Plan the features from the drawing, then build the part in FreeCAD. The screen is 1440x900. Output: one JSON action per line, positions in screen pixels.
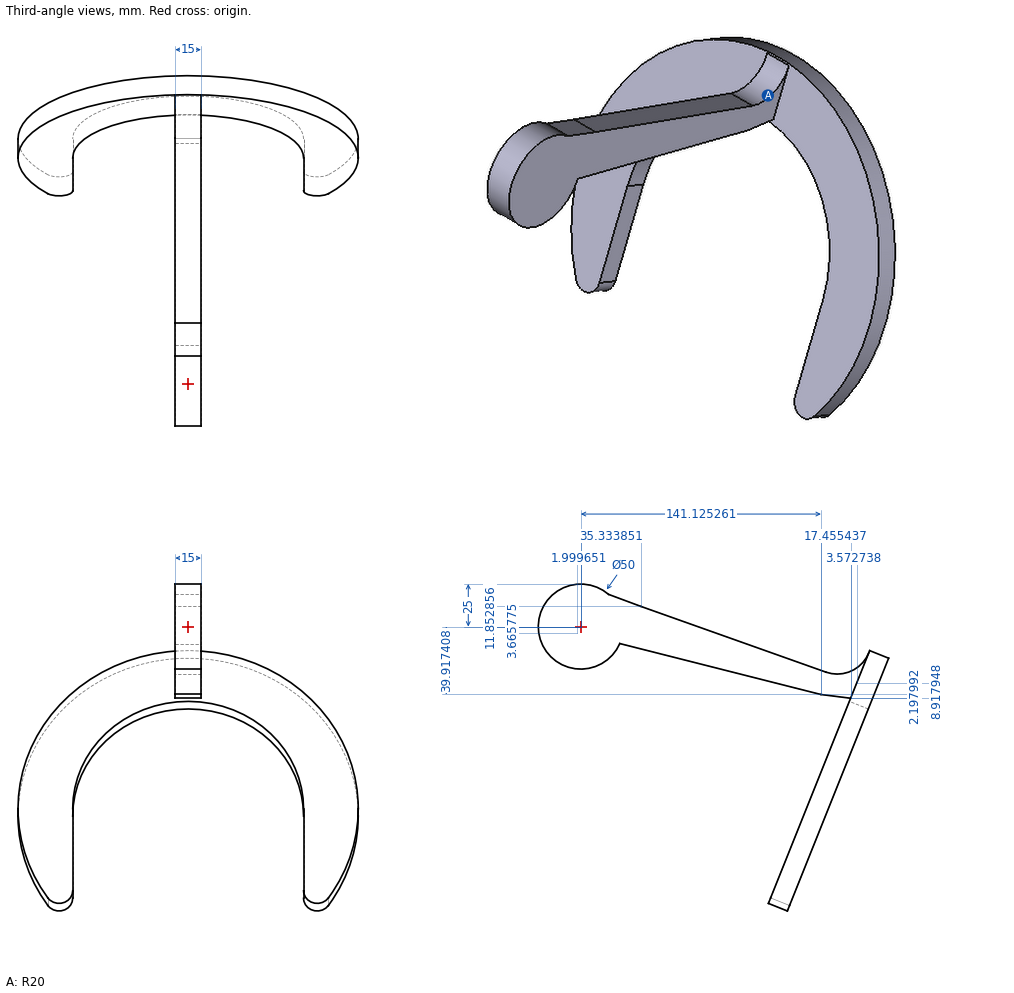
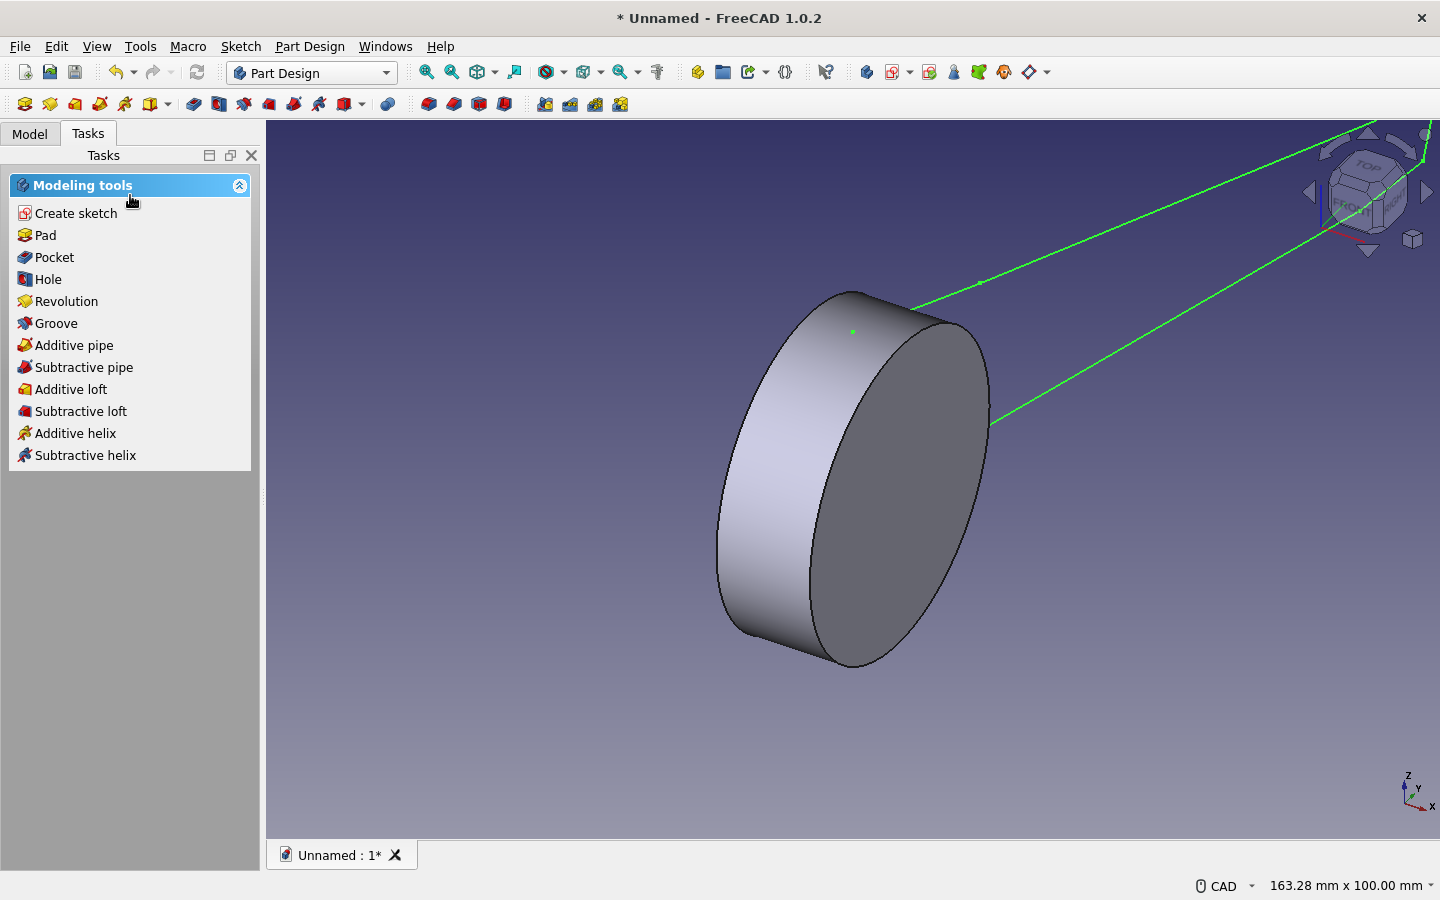
{"action": "left_click", "coordinate": [25, 104]}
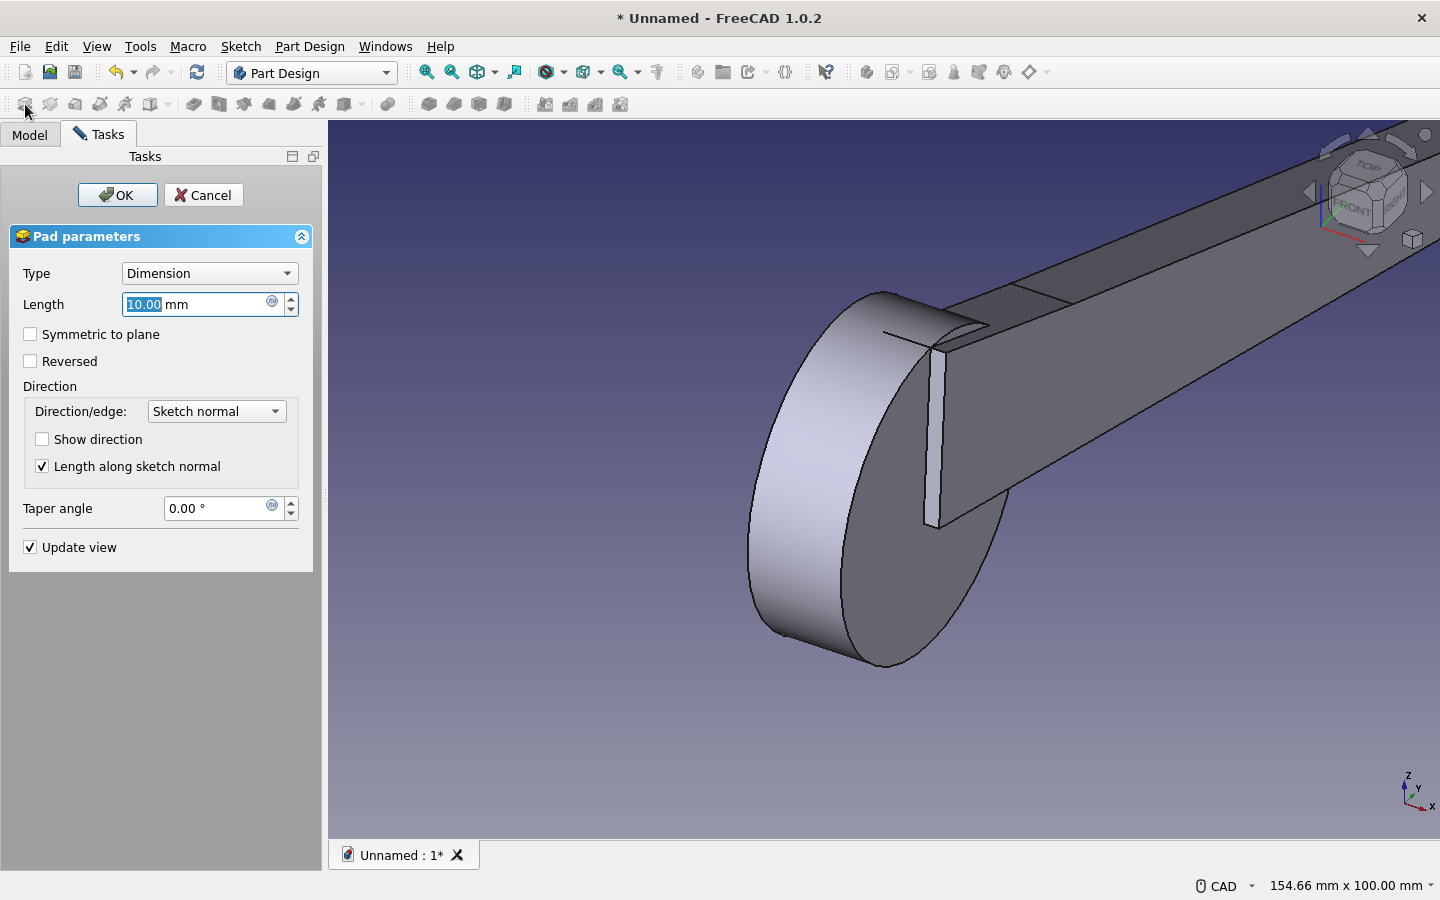
{"action": "type", "text": "15"}
{"action": "key", "text": "Tab"}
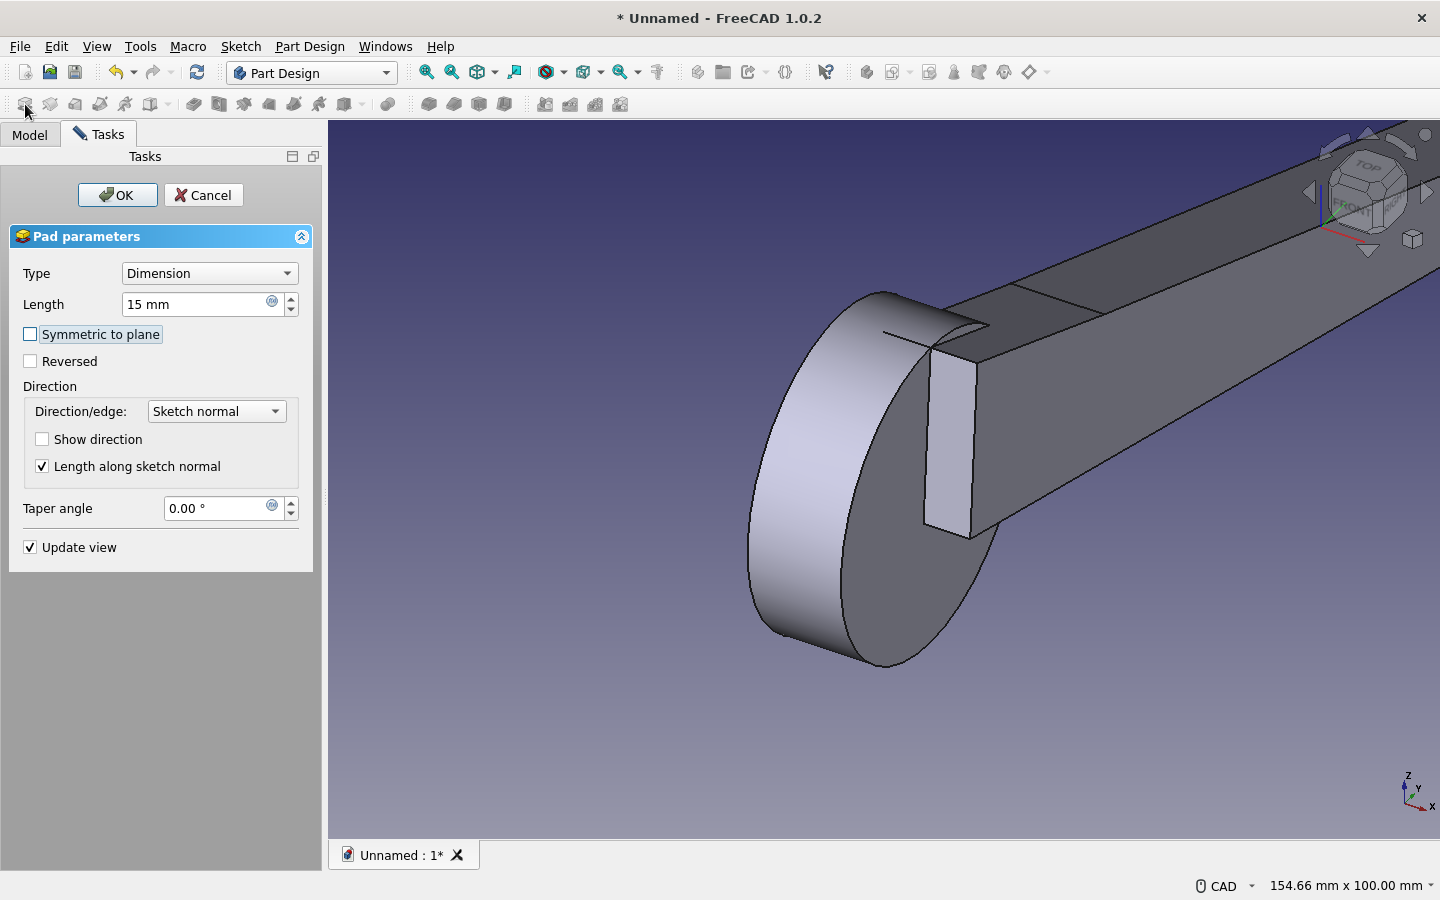
{"action": "left_click", "coordinate": [31, 334]}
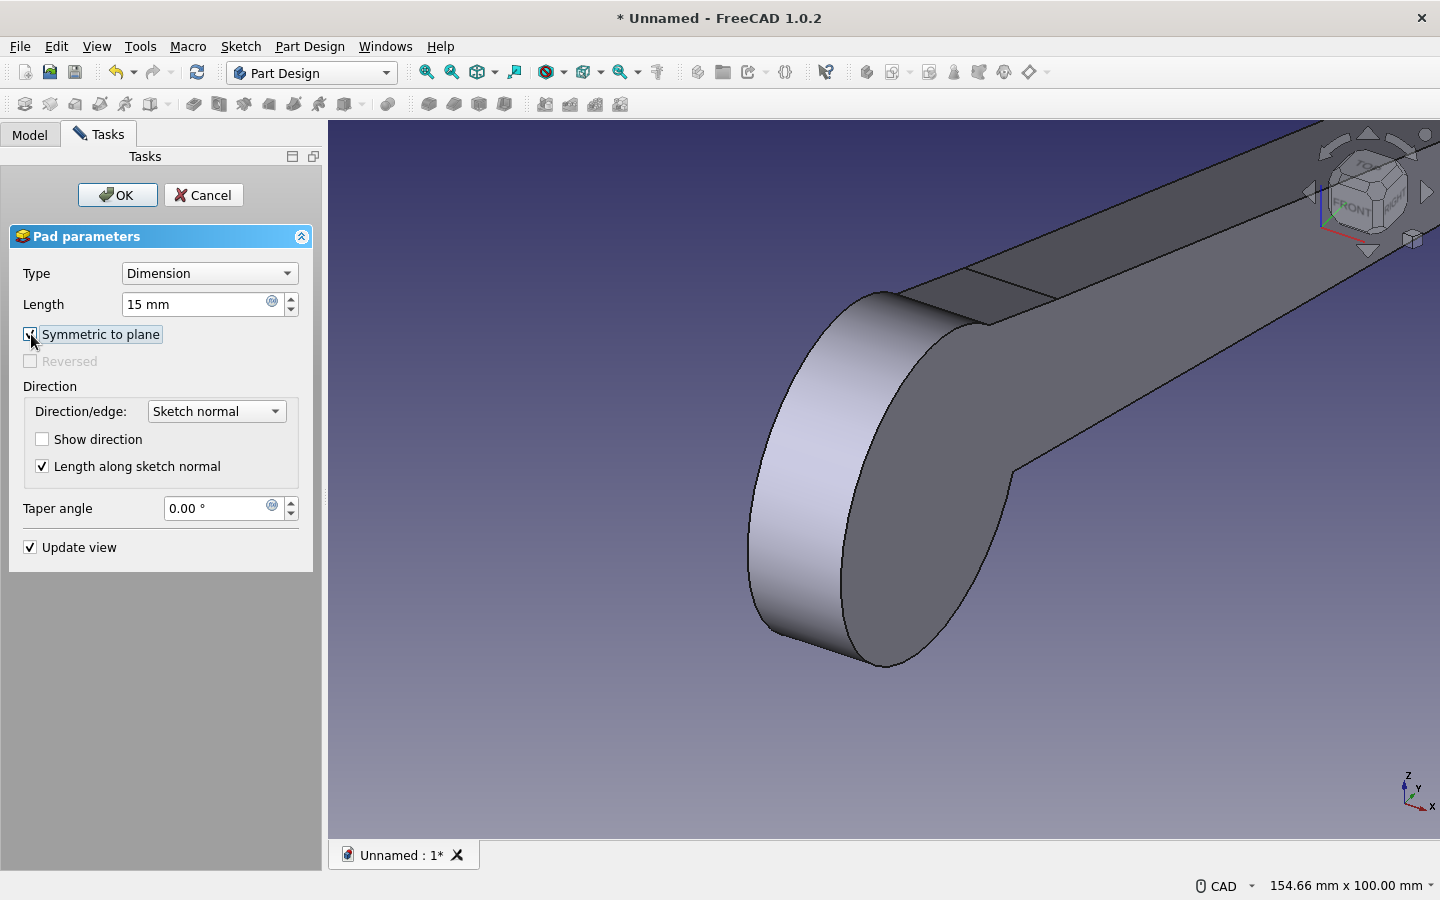
{"action": "left_click", "coordinate": [118, 195]}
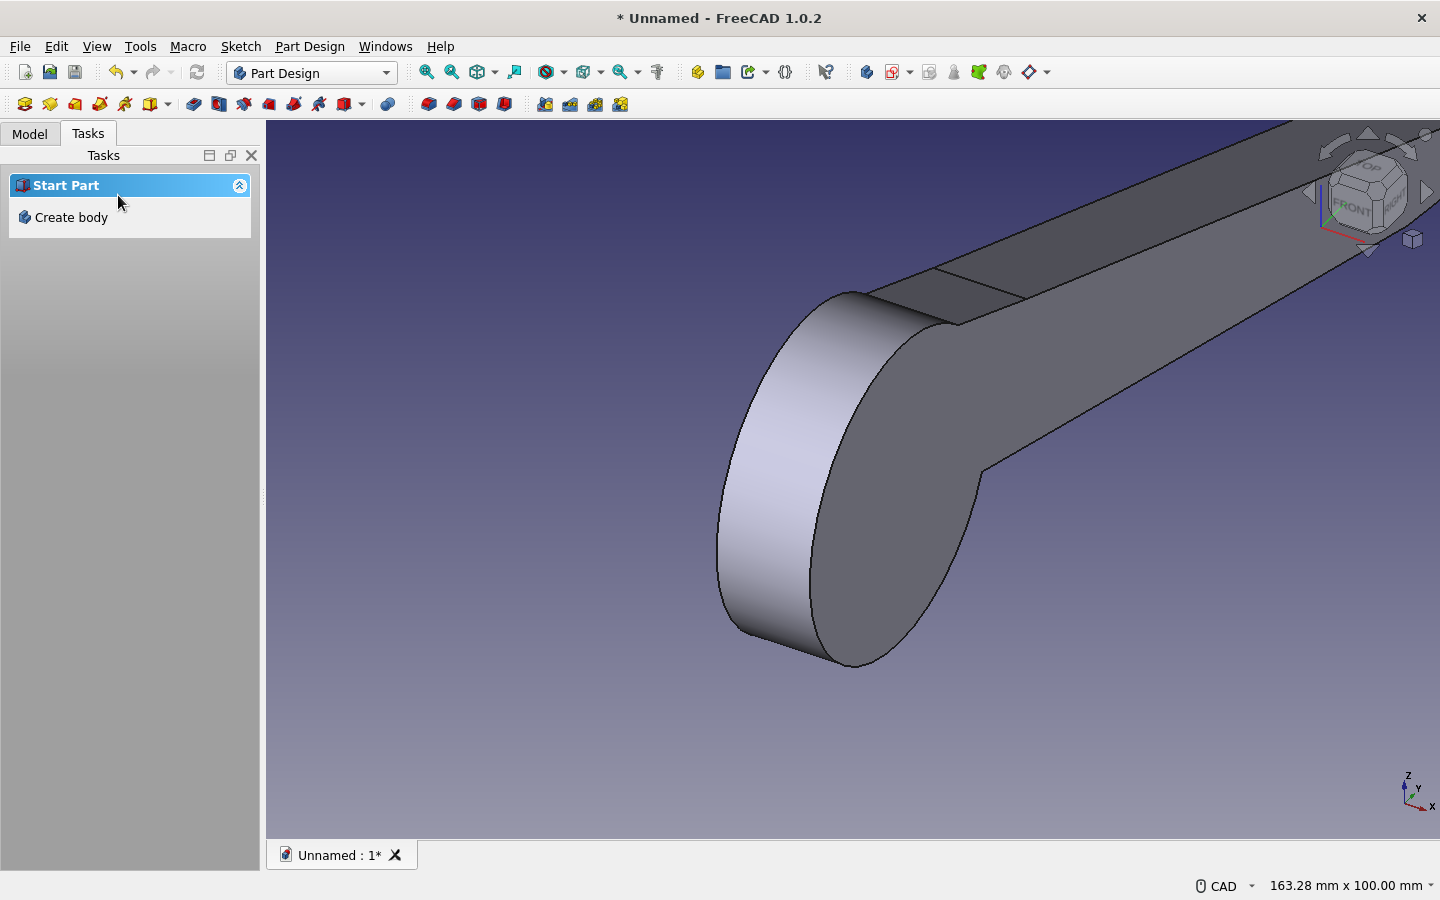
{"action": "left_click", "coordinate": [427, 72]}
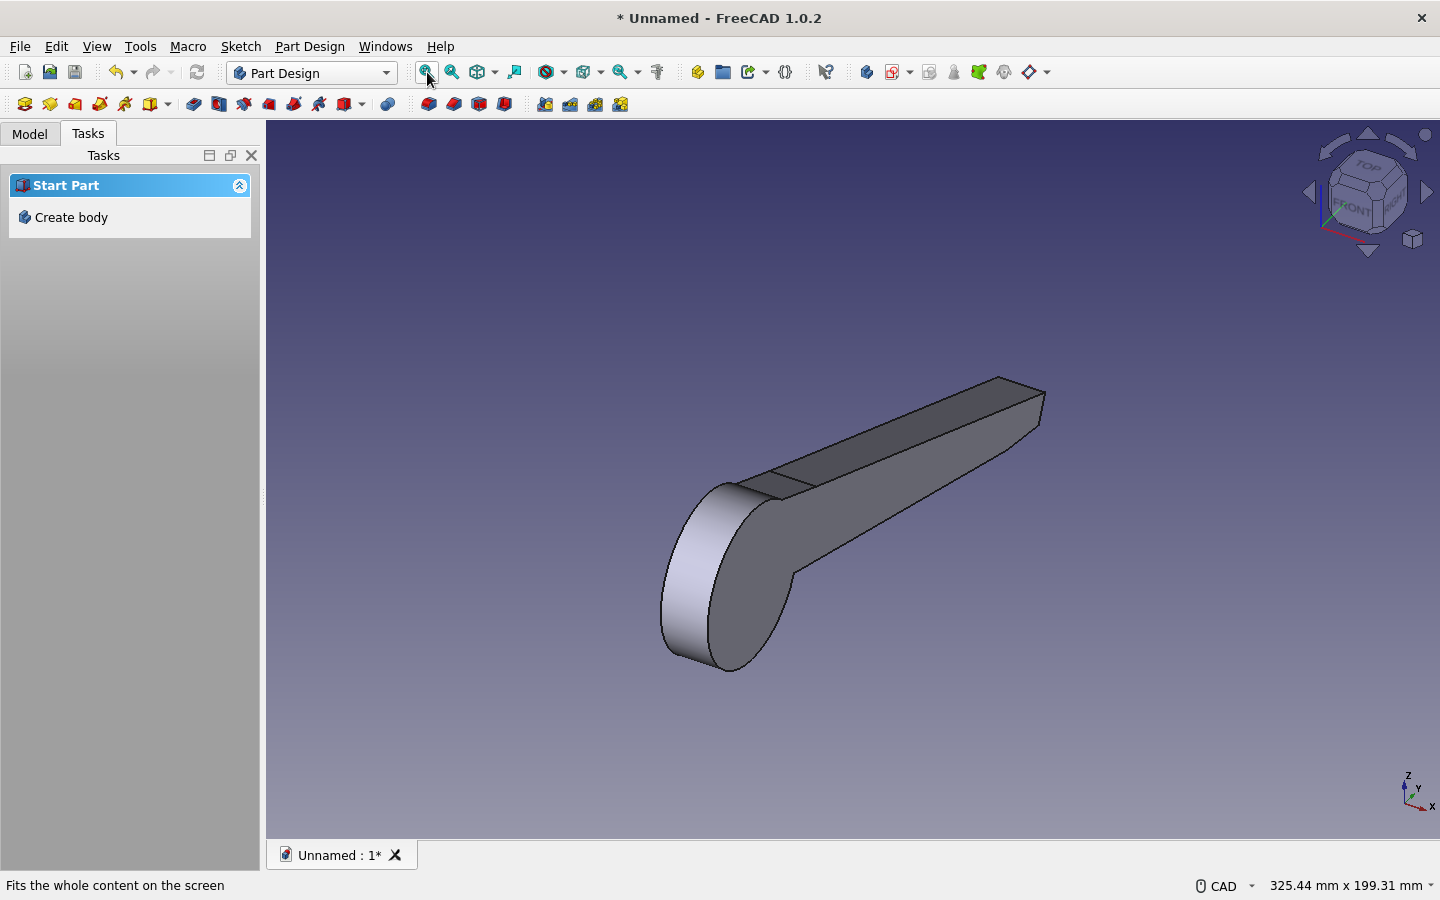
{"action": "key", "text": "4"}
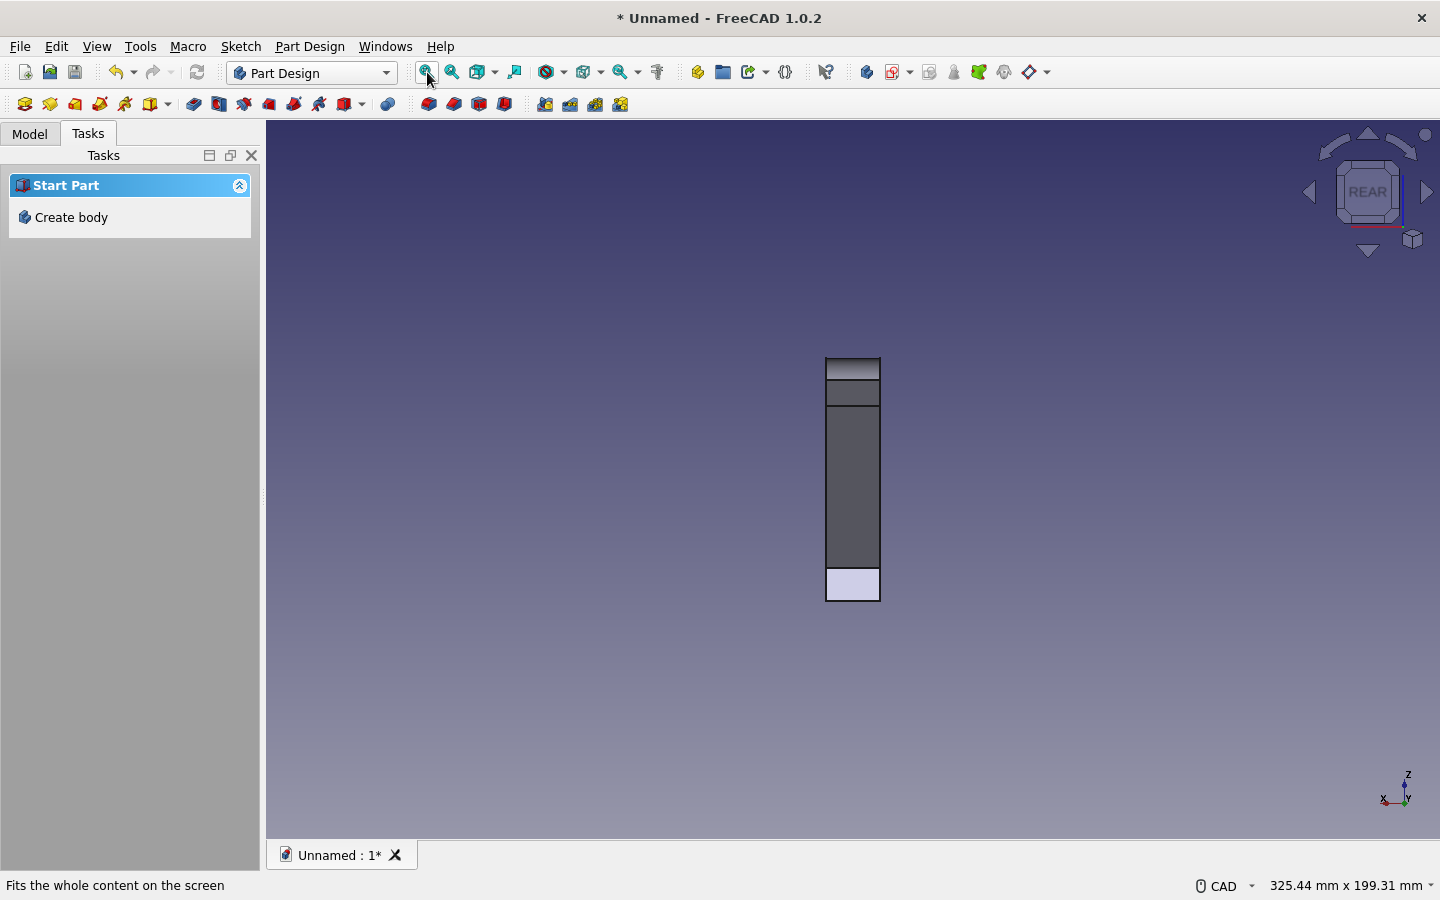
{"action": "left_click", "coordinate": [427, 72]}